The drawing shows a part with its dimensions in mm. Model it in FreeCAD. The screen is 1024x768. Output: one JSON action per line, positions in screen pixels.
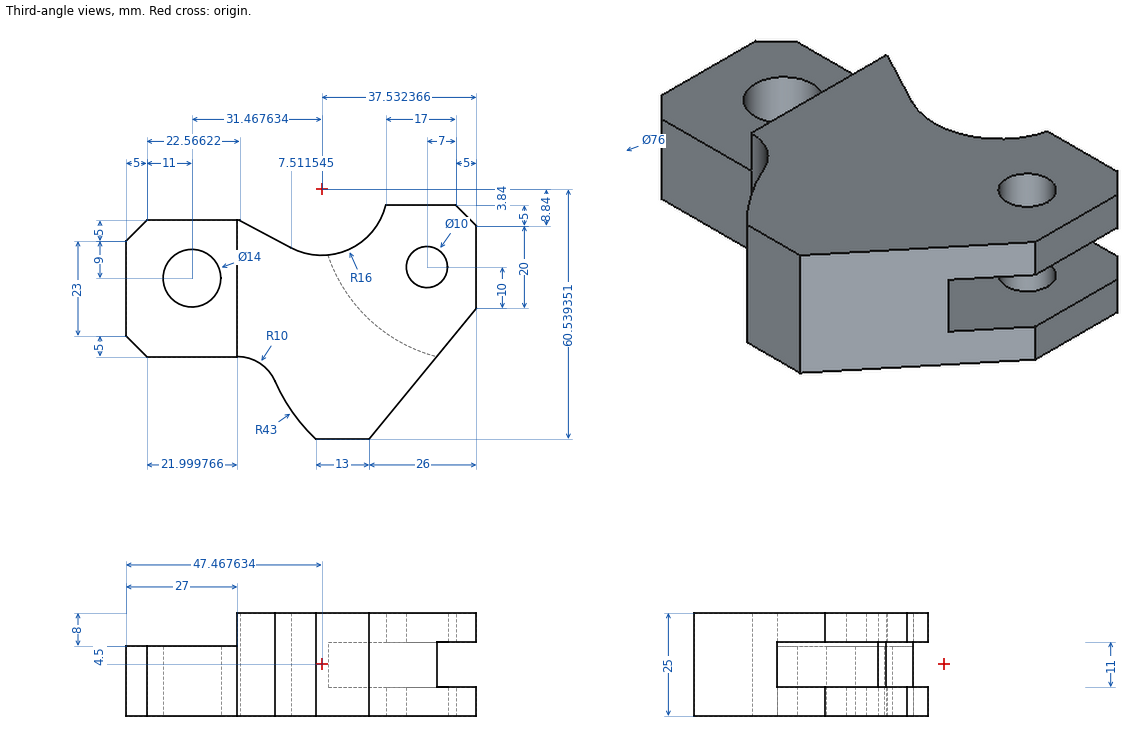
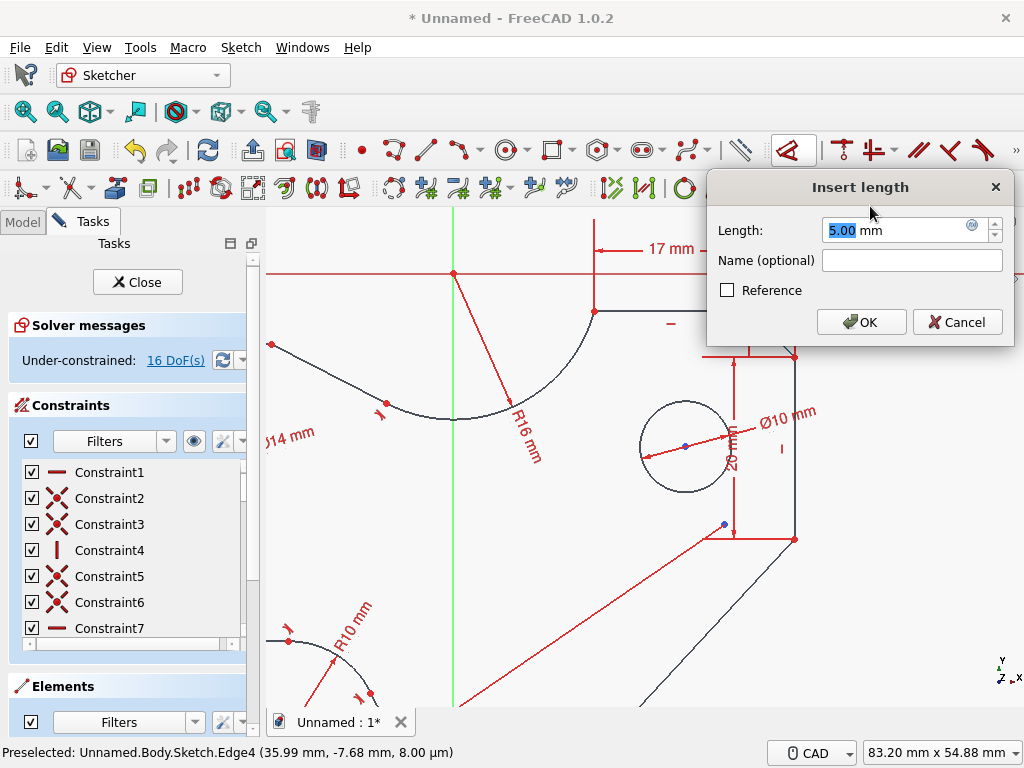
{"action": "type", "text": "5"}
{"action": "key", "text": "Return"}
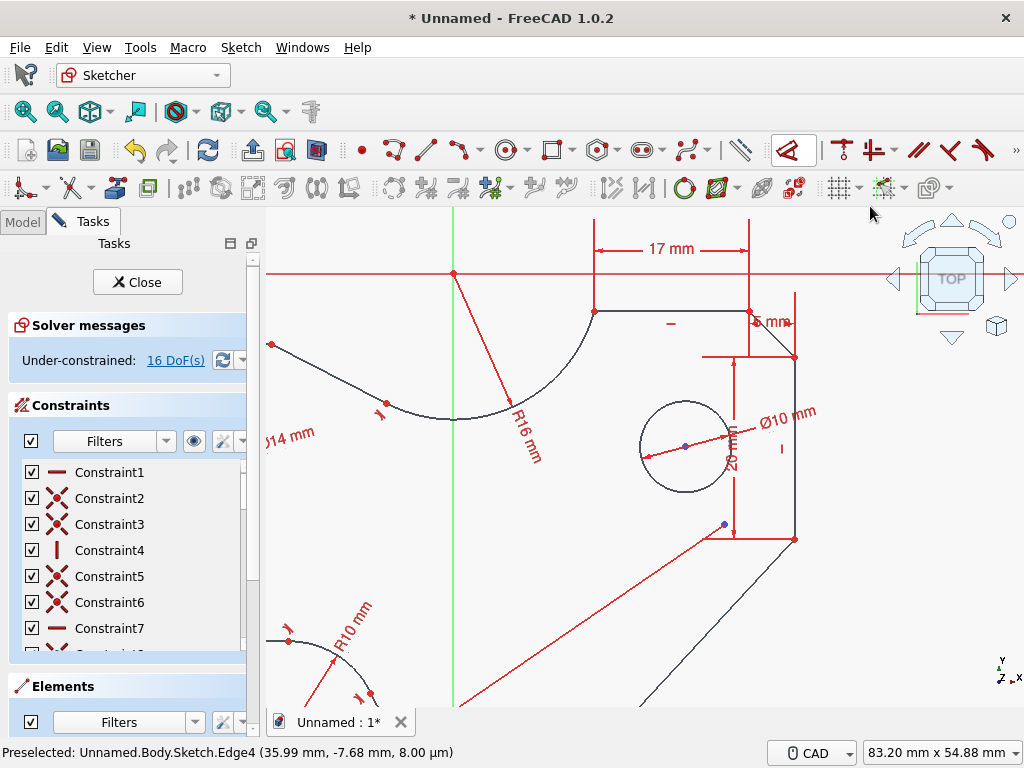
{"action": "left_click", "coordinate": [781, 343]}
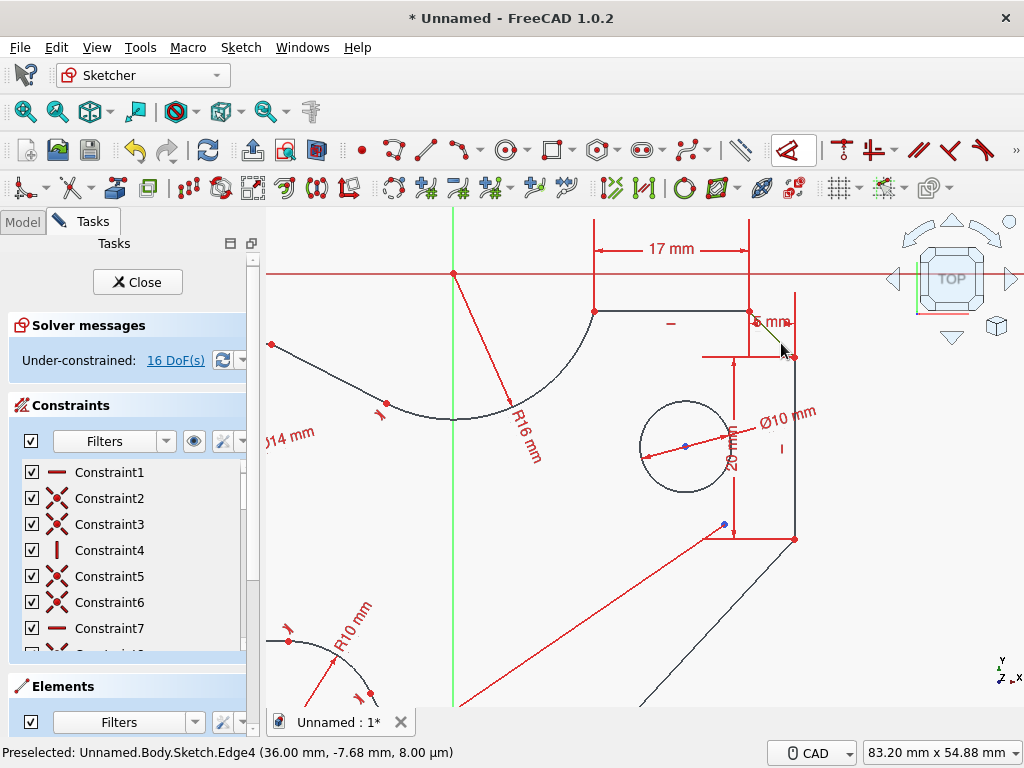
{"action": "left_click", "coordinate": [810, 150]}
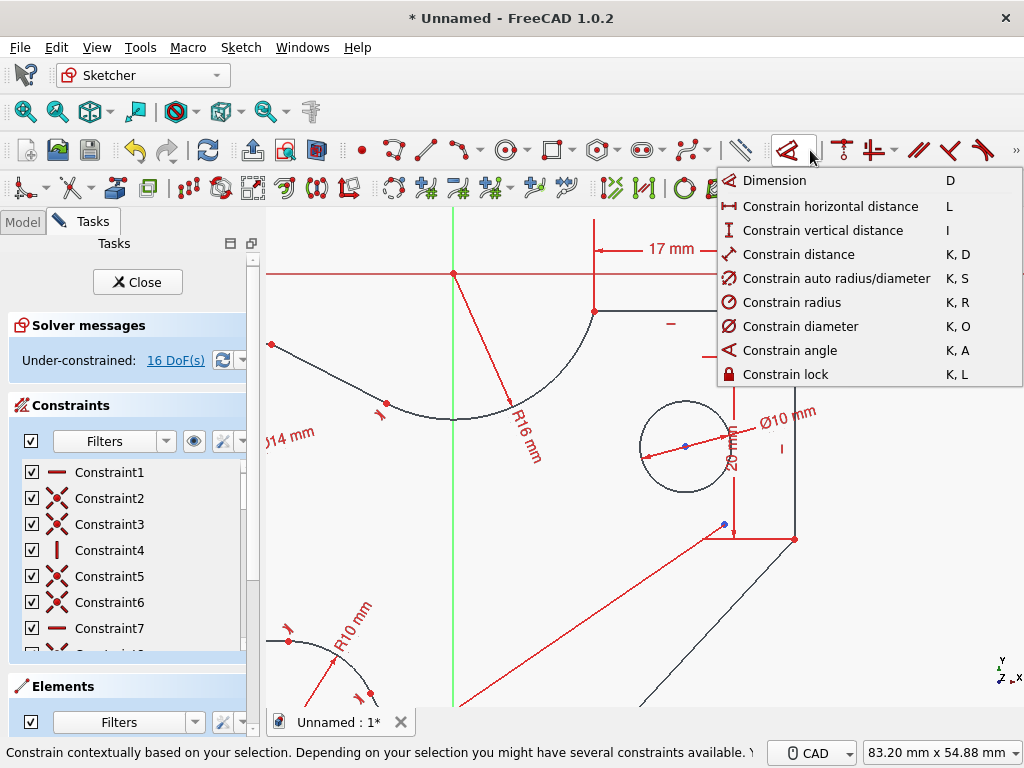
{"action": "left_click", "coordinate": [870, 230]}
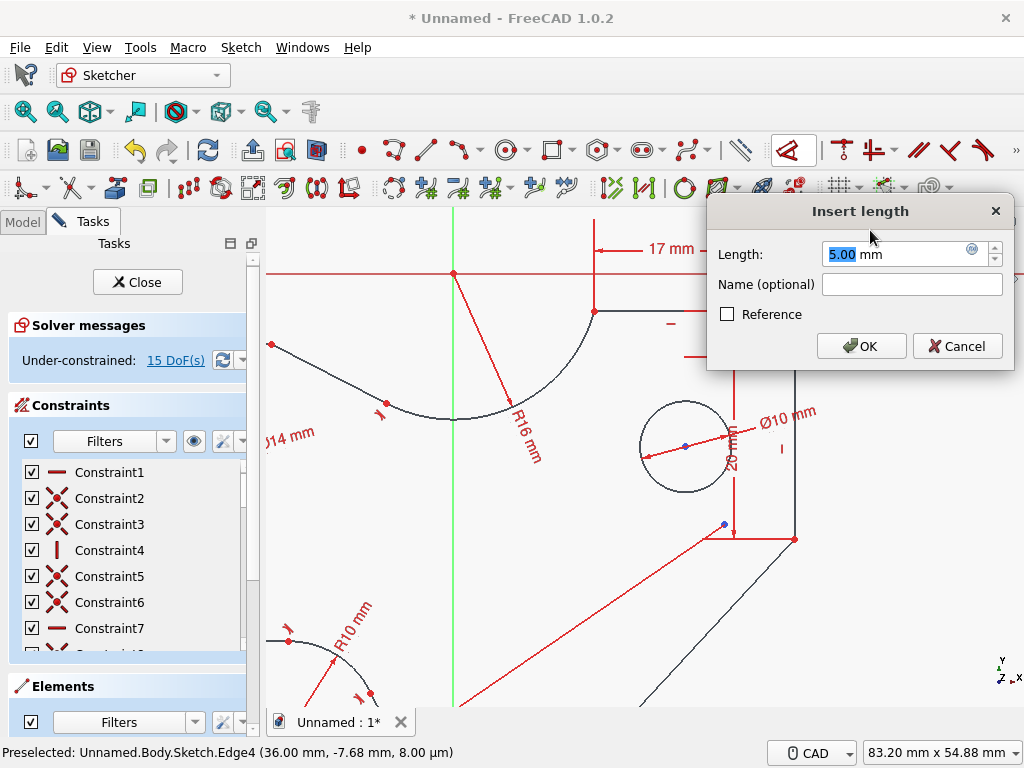
{"action": "type", "text": "5"}
{"action": "key", "text": "Return"}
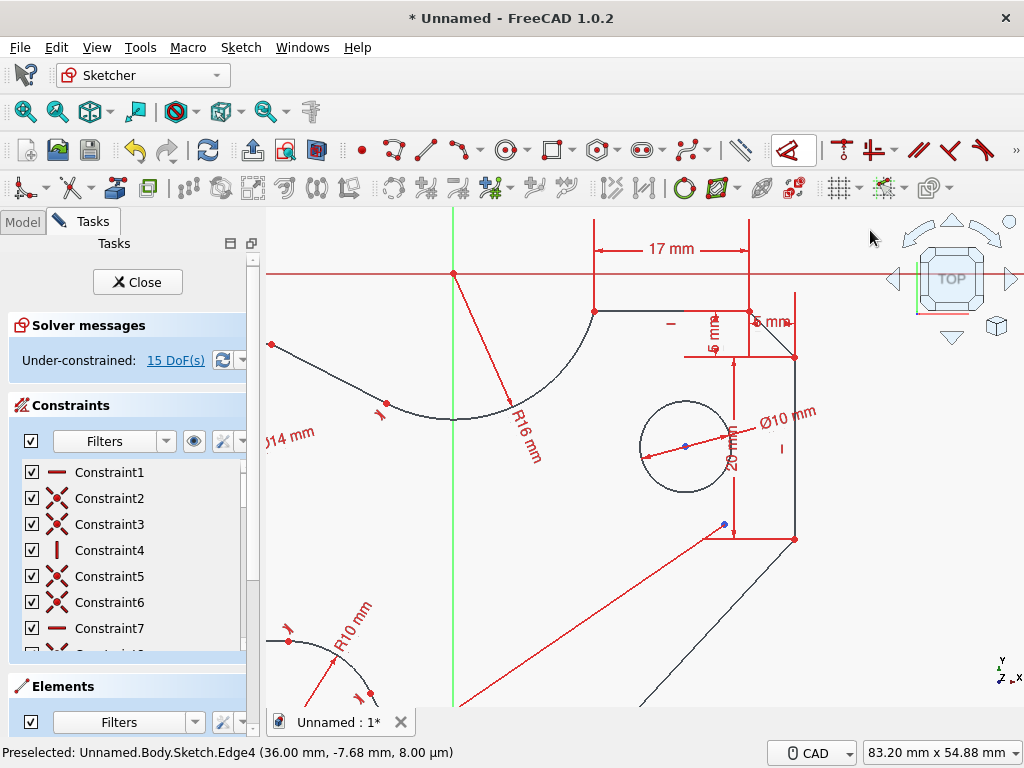
{"action": "scroll", "coordinate": [781, 344], "scroll_direction": "down", "scroll_amount": 3}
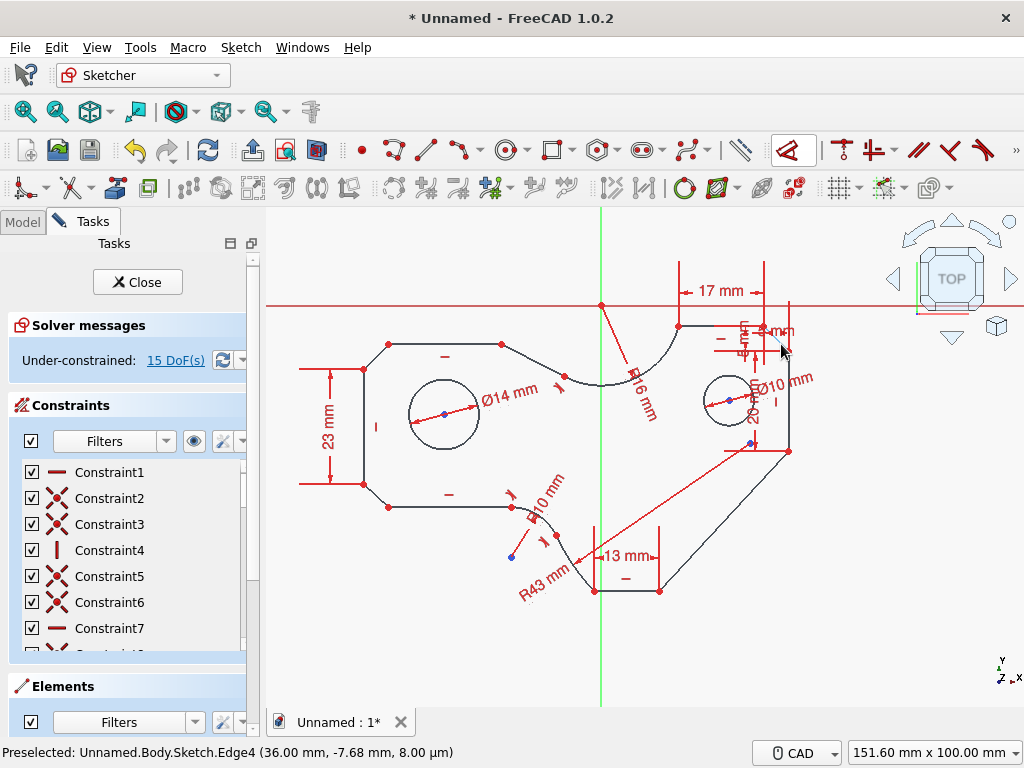
{"action": "scroll", "coordinate": [381, 352], "scroll_direction": "up", "scroll_amount": 3}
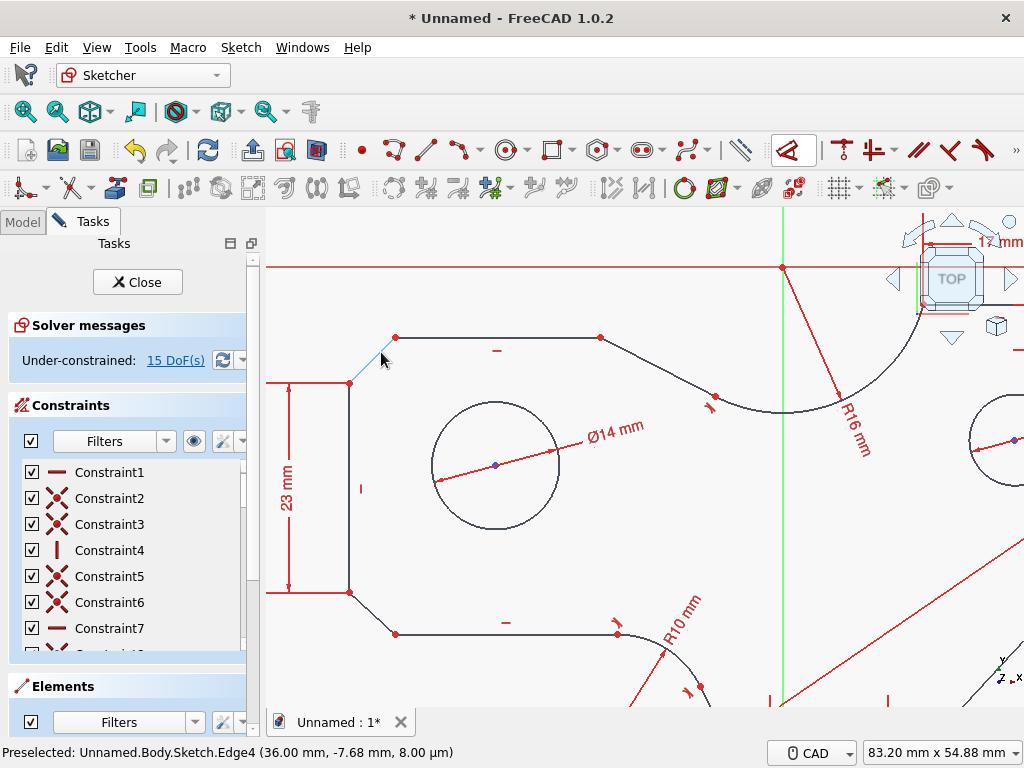
{"action": "left_click", "coordinate": [381, 351]}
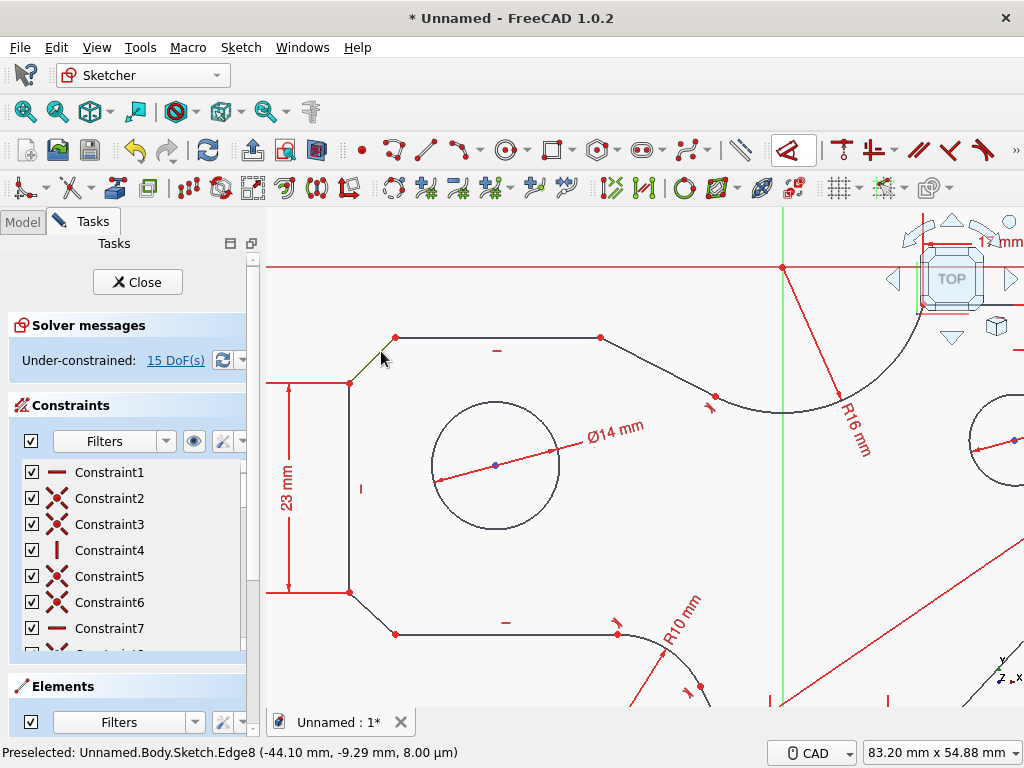
{"action": "key", "text": "l"}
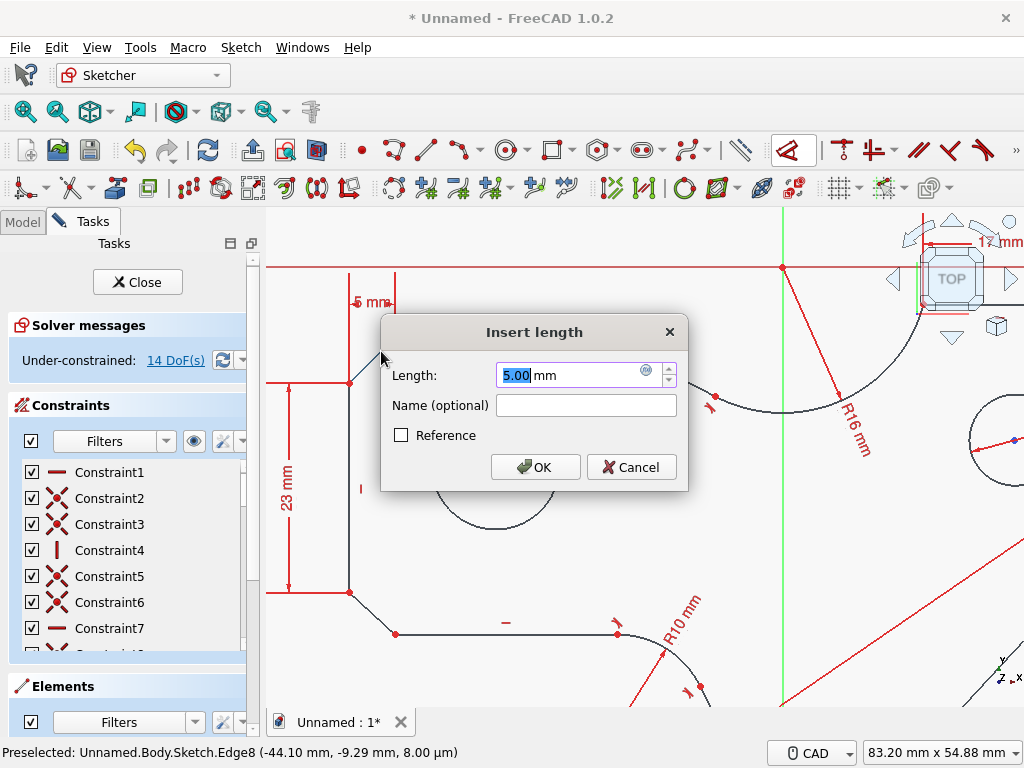
{"action": "type", "text": "5"}
{"action": "key", "text": "Return"}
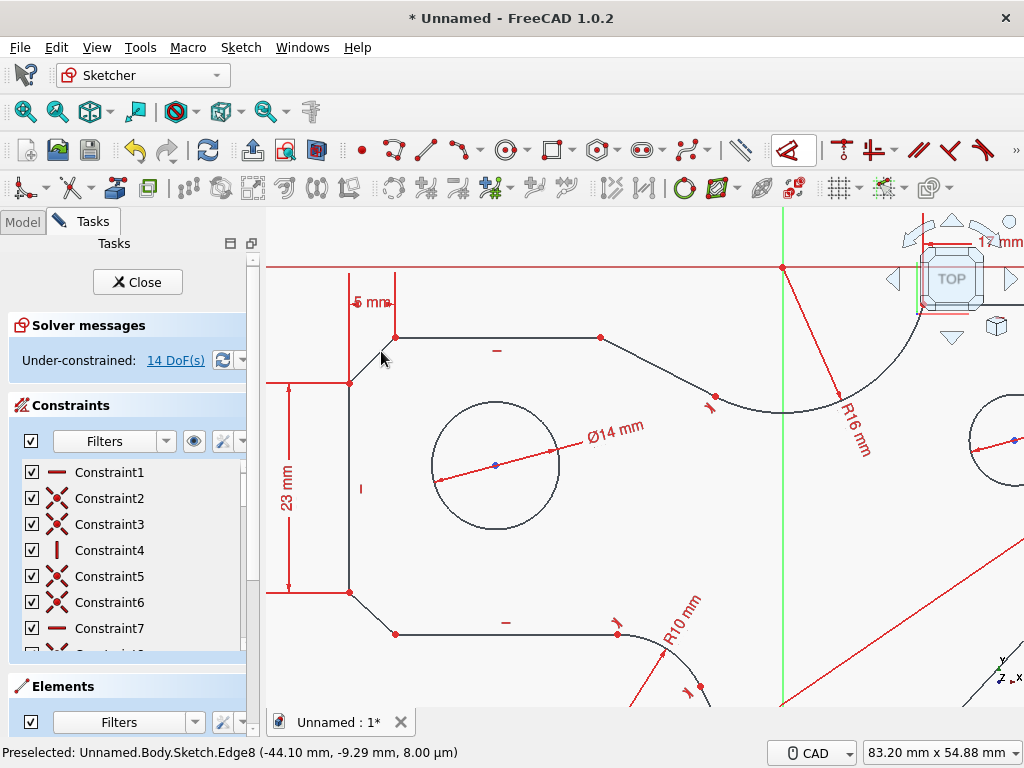
{"action": "left_click", "coordinate": [381, 351]}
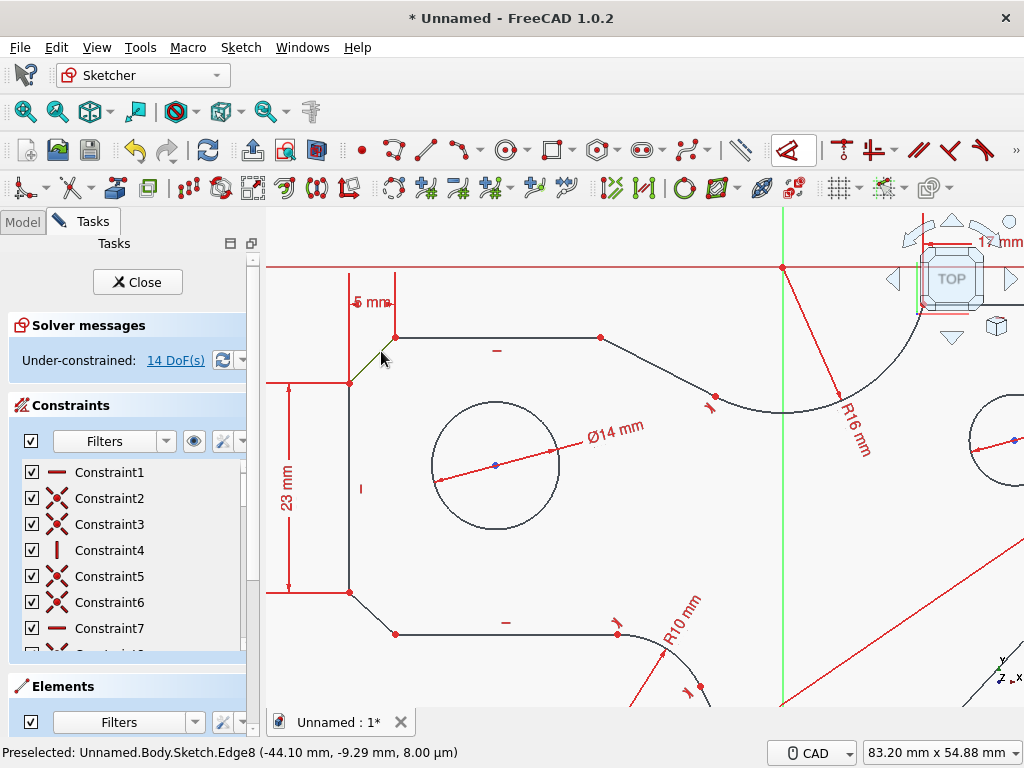
{"action": "left_click", "coordinate": [810, 150]}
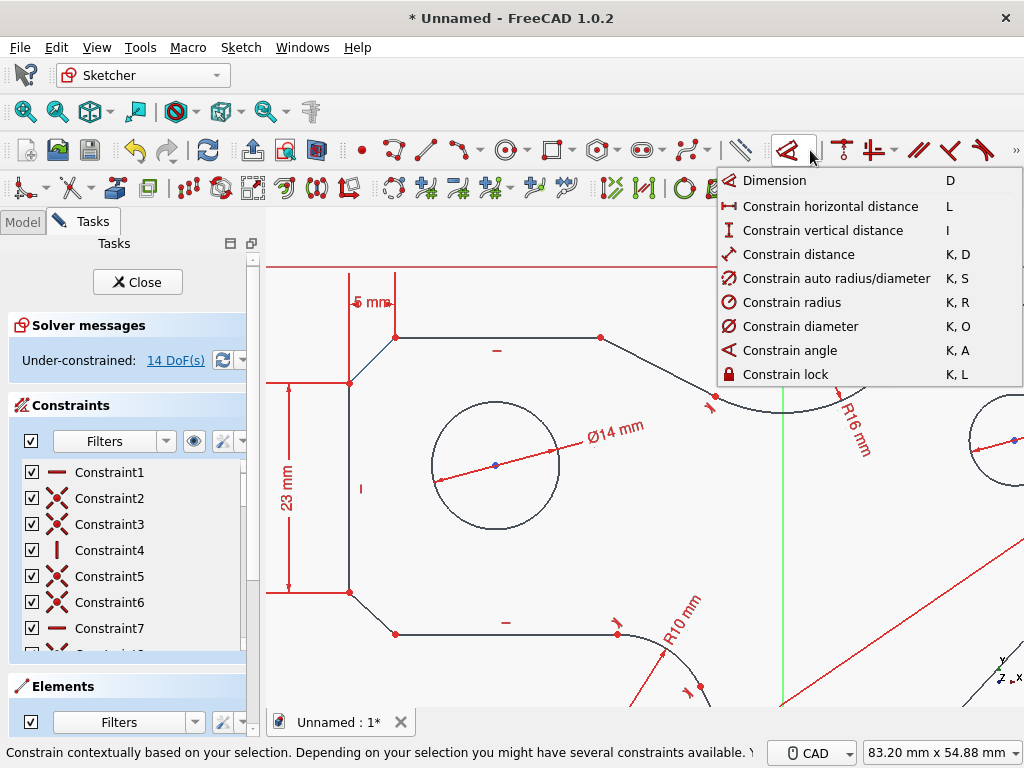
{"action": "left_click", "coordinate": [870, 230]}